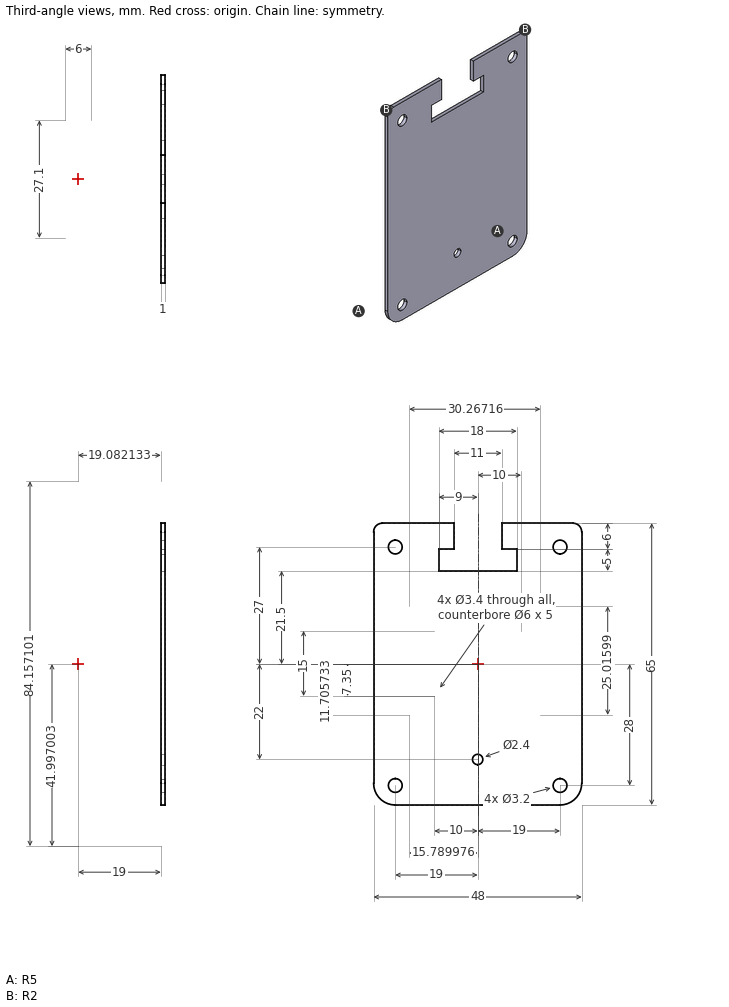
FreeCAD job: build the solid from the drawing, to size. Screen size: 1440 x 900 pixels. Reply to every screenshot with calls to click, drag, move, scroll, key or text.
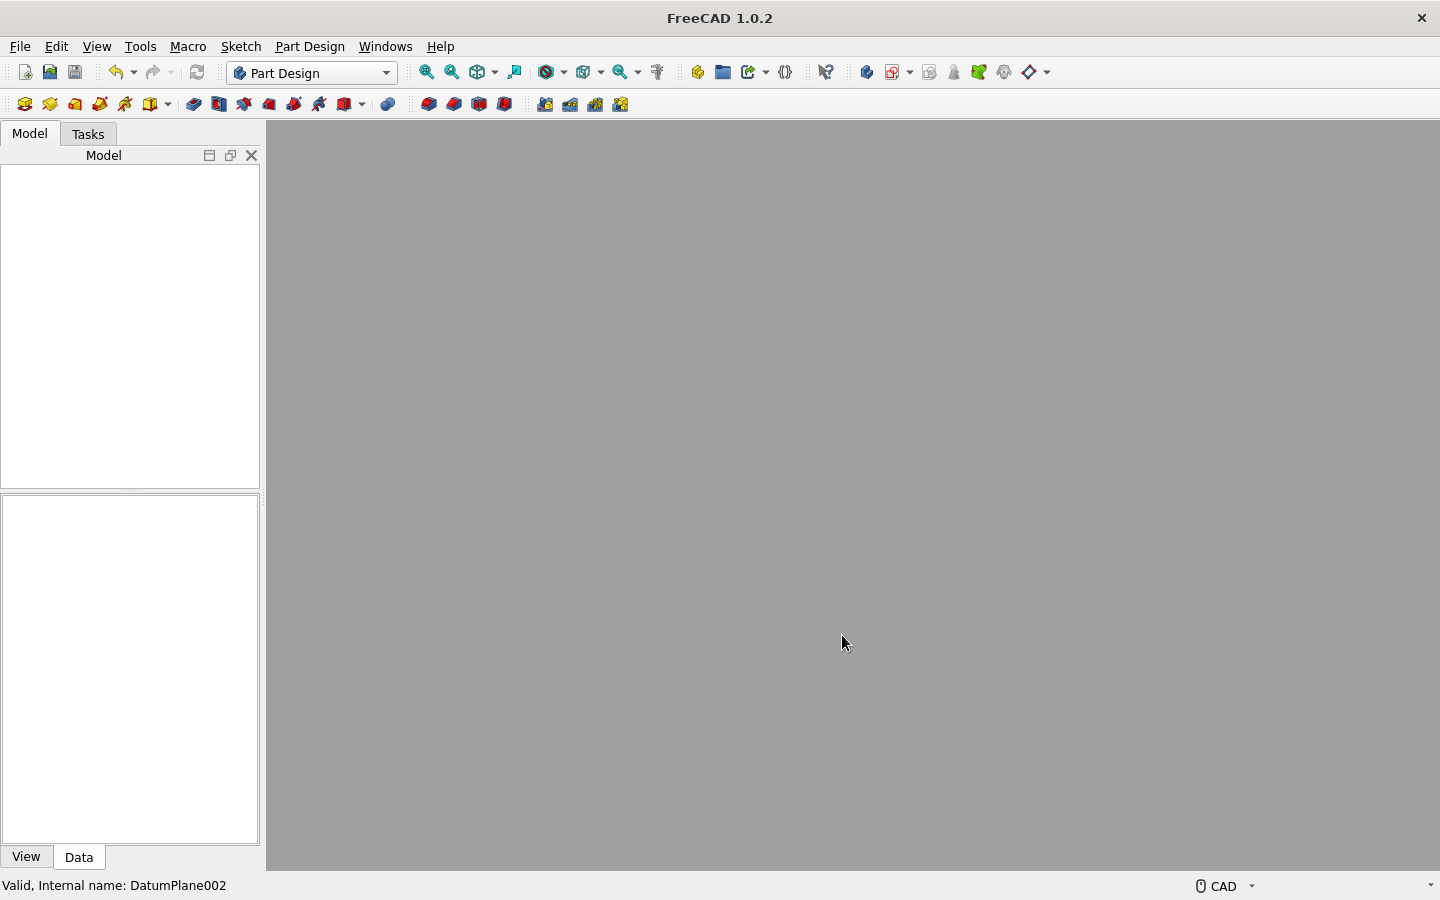
key(ctrl+n)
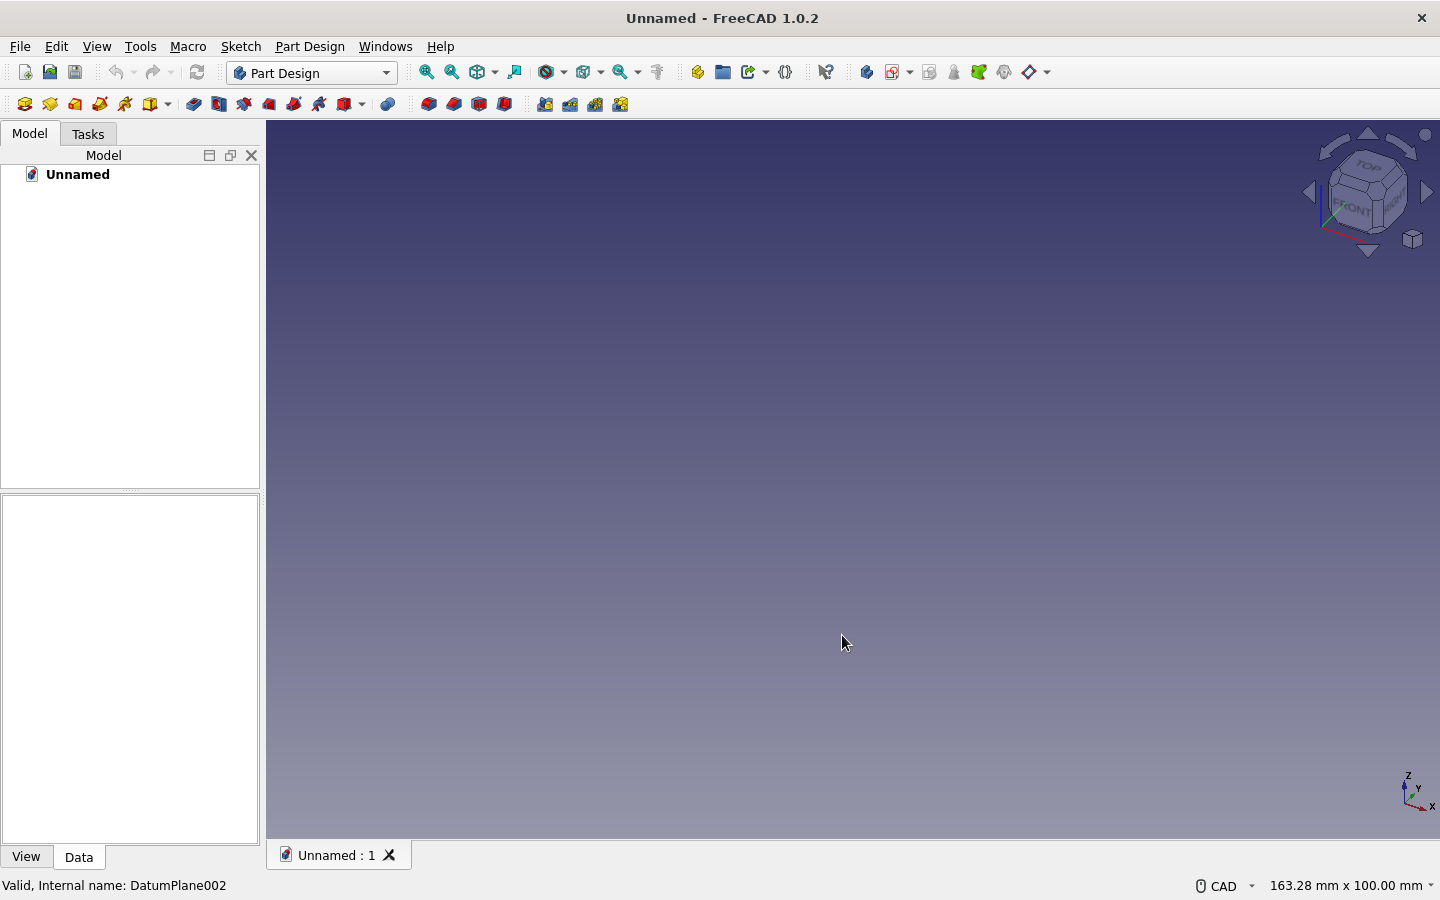
click(892, 72)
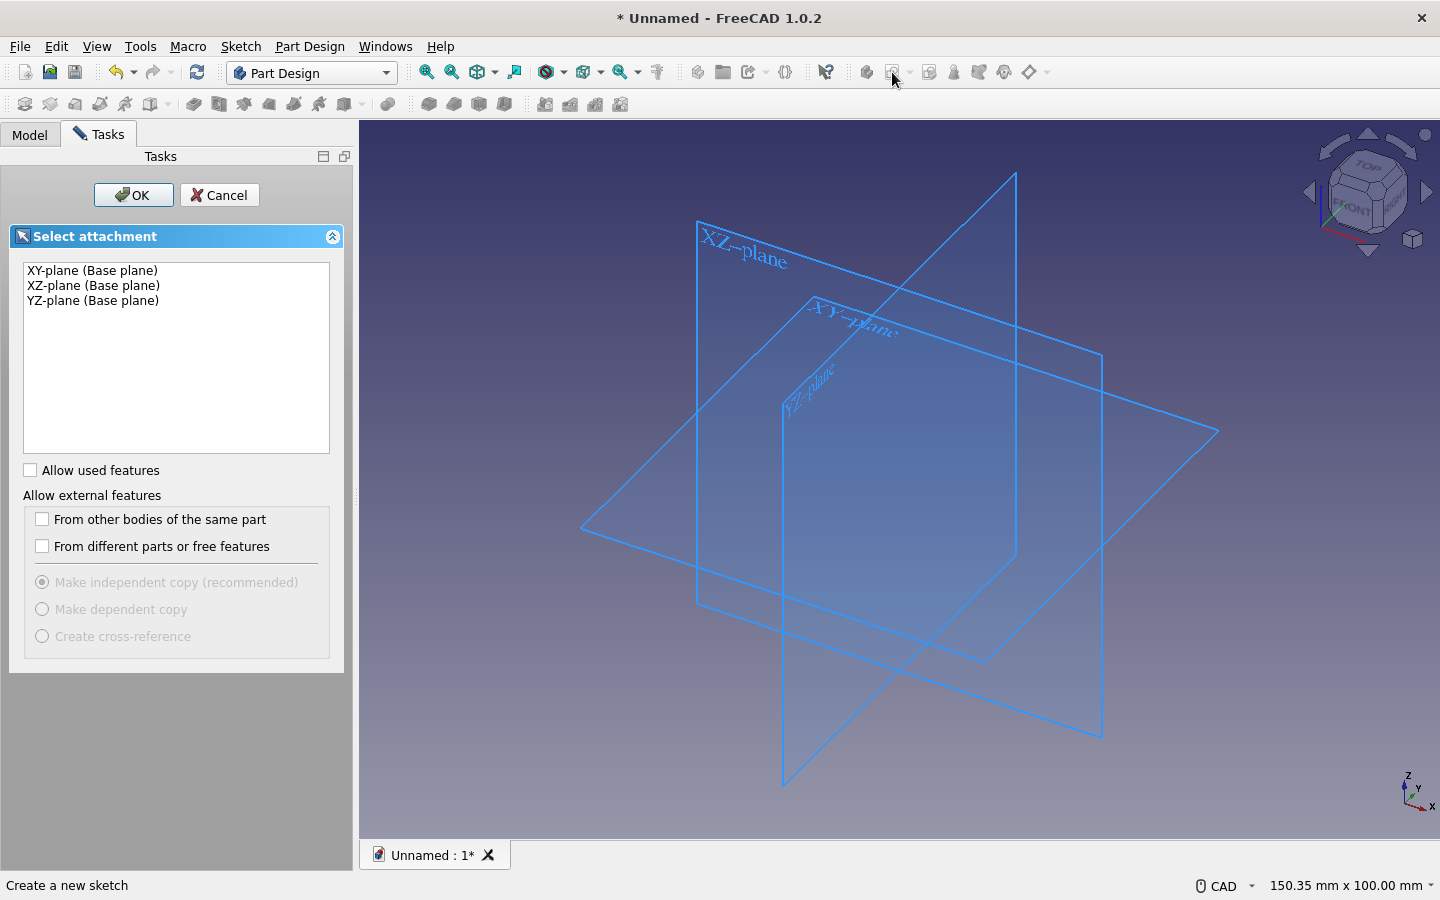
click(84, 300)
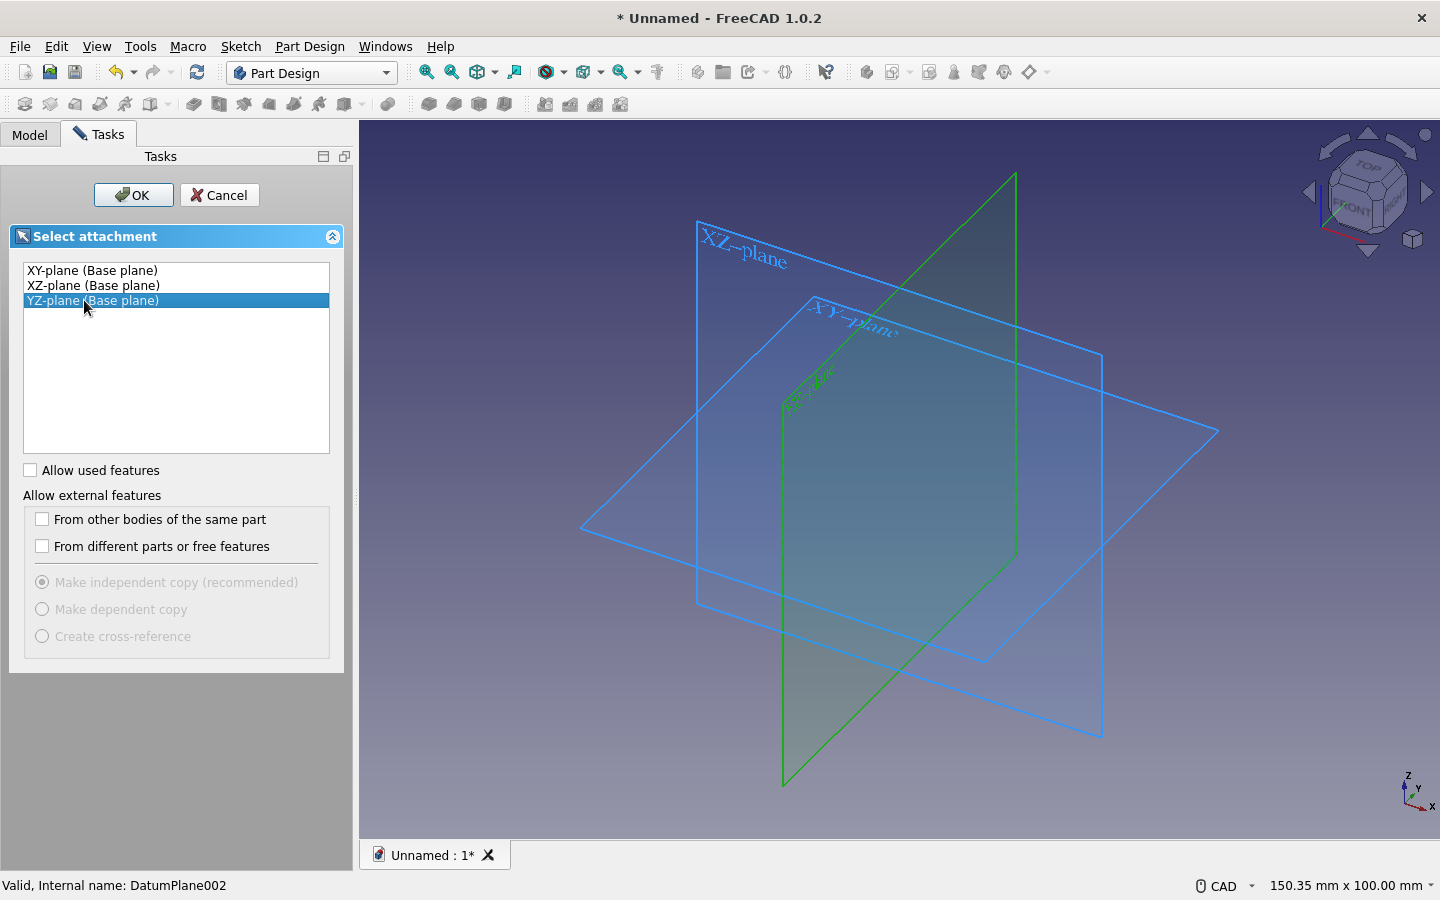
click(134, 195)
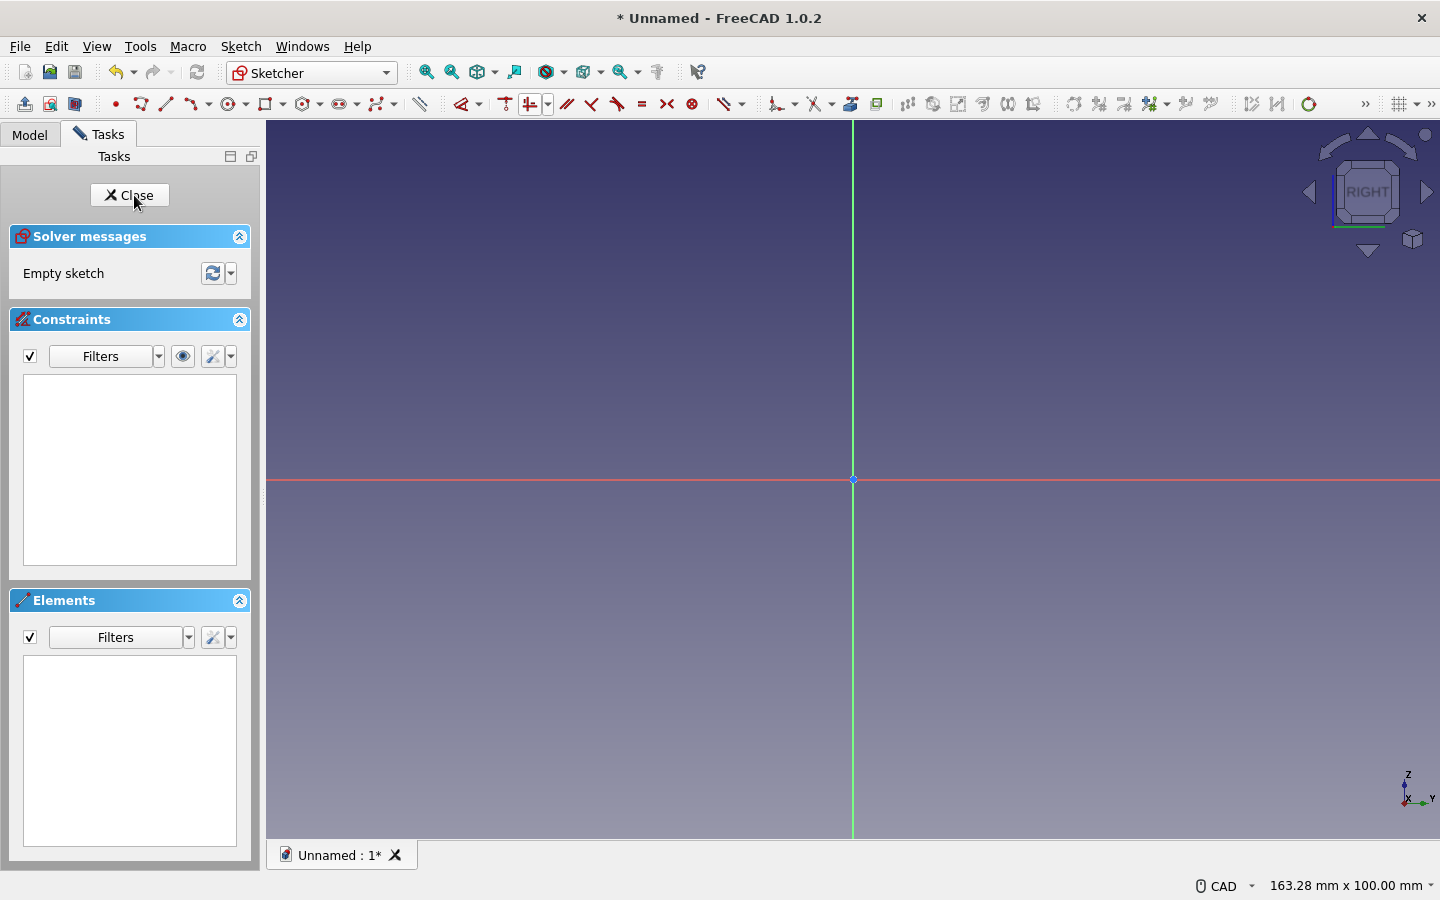
click(282, 104)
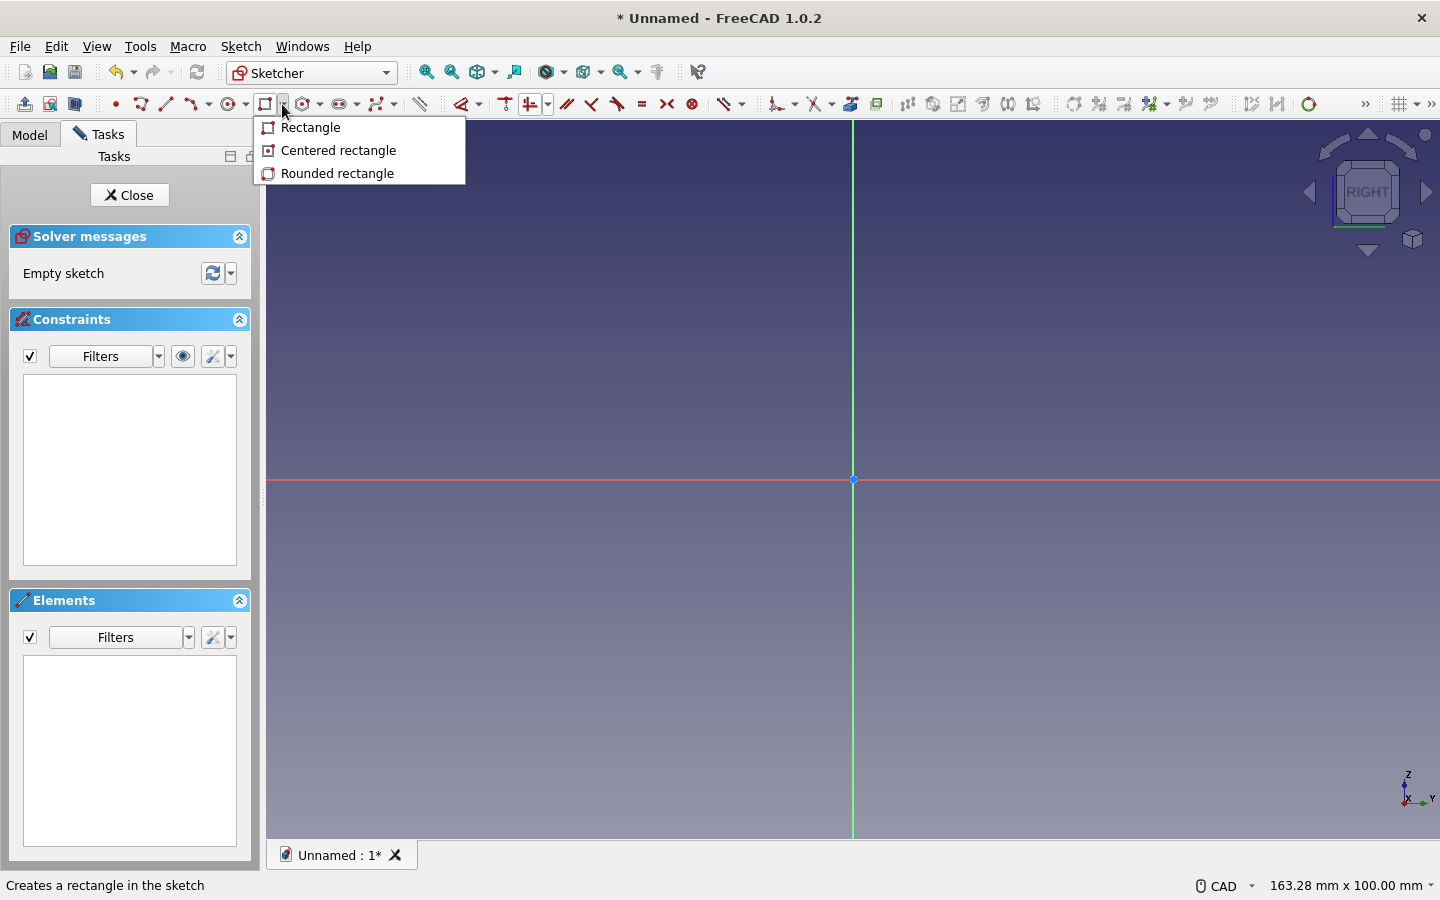
click(360, 150)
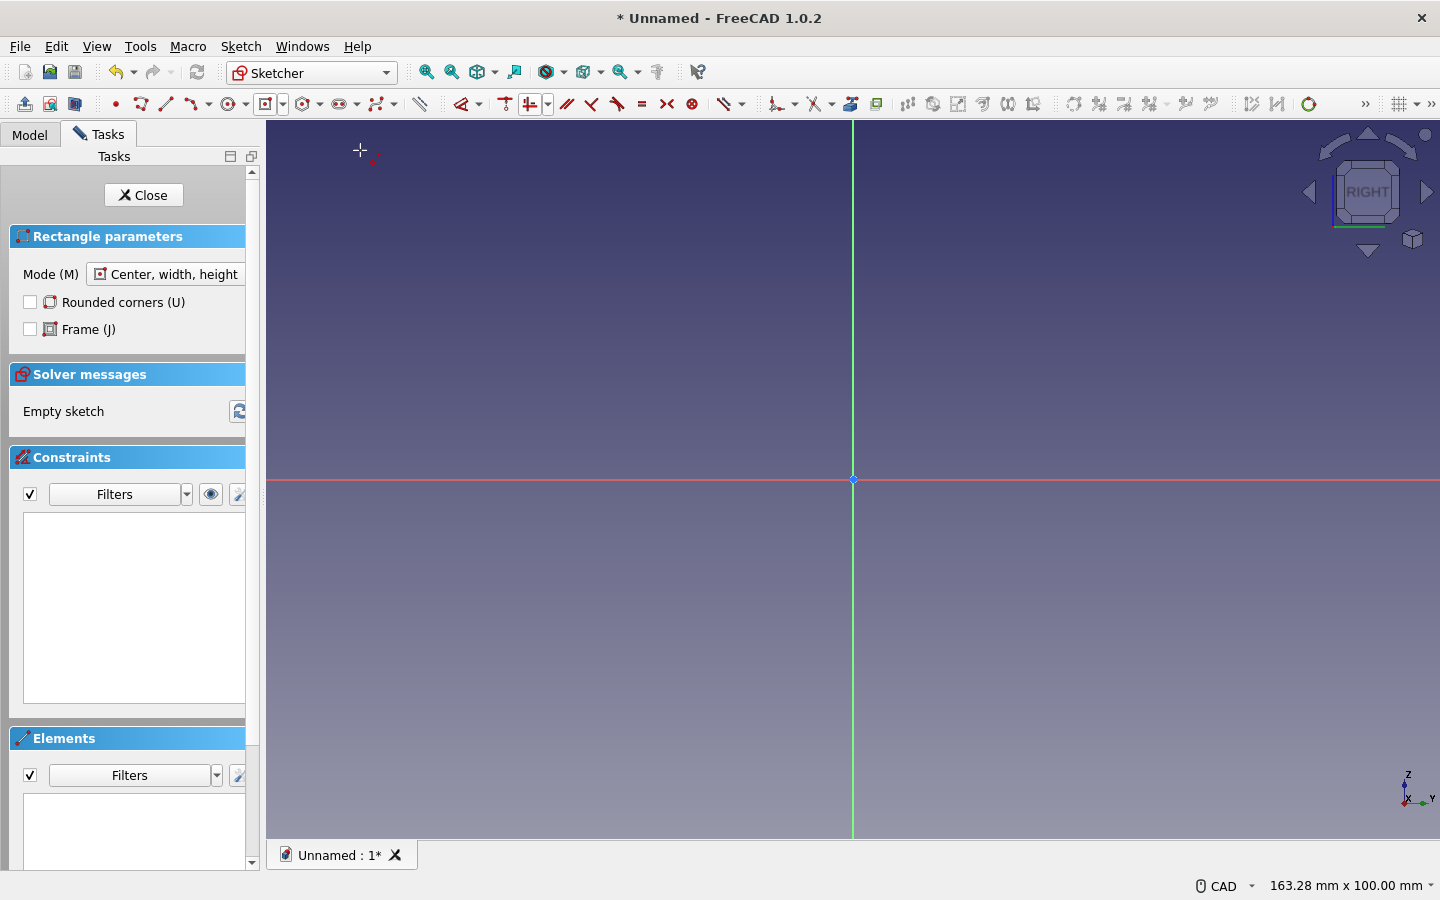
click(853, 480)
move(1026, 246)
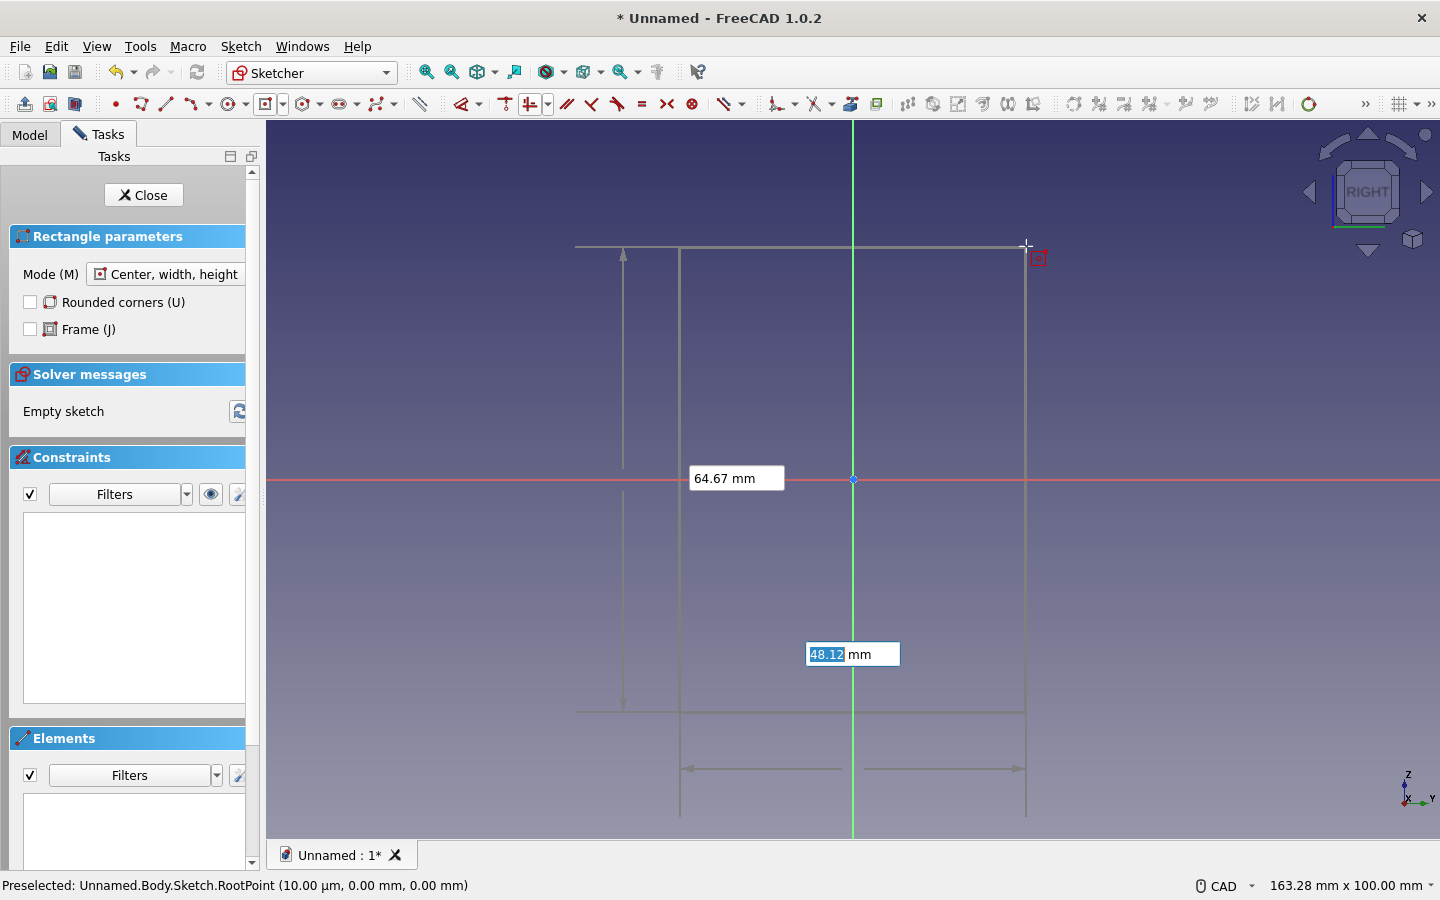
text(48)
key(Tab)
text(65)
key(Return)
key(Escape)